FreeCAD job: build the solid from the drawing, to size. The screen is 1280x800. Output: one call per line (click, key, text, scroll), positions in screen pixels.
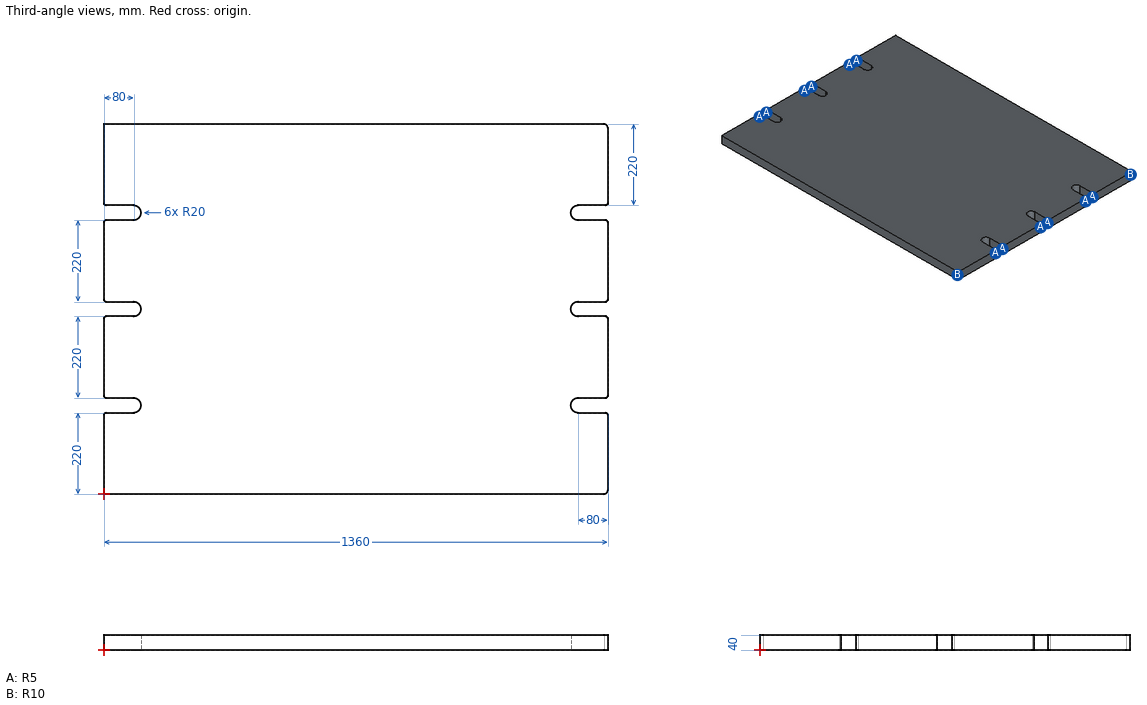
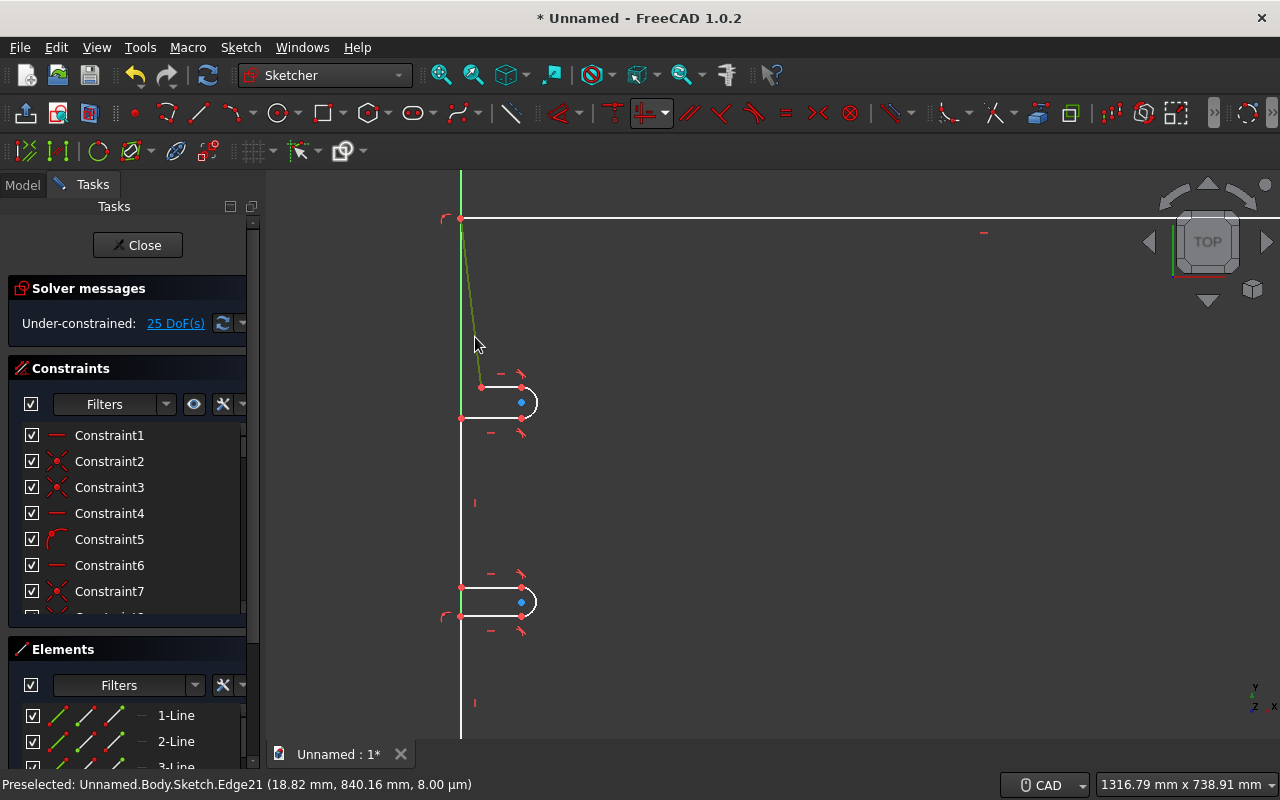
click(668, 114)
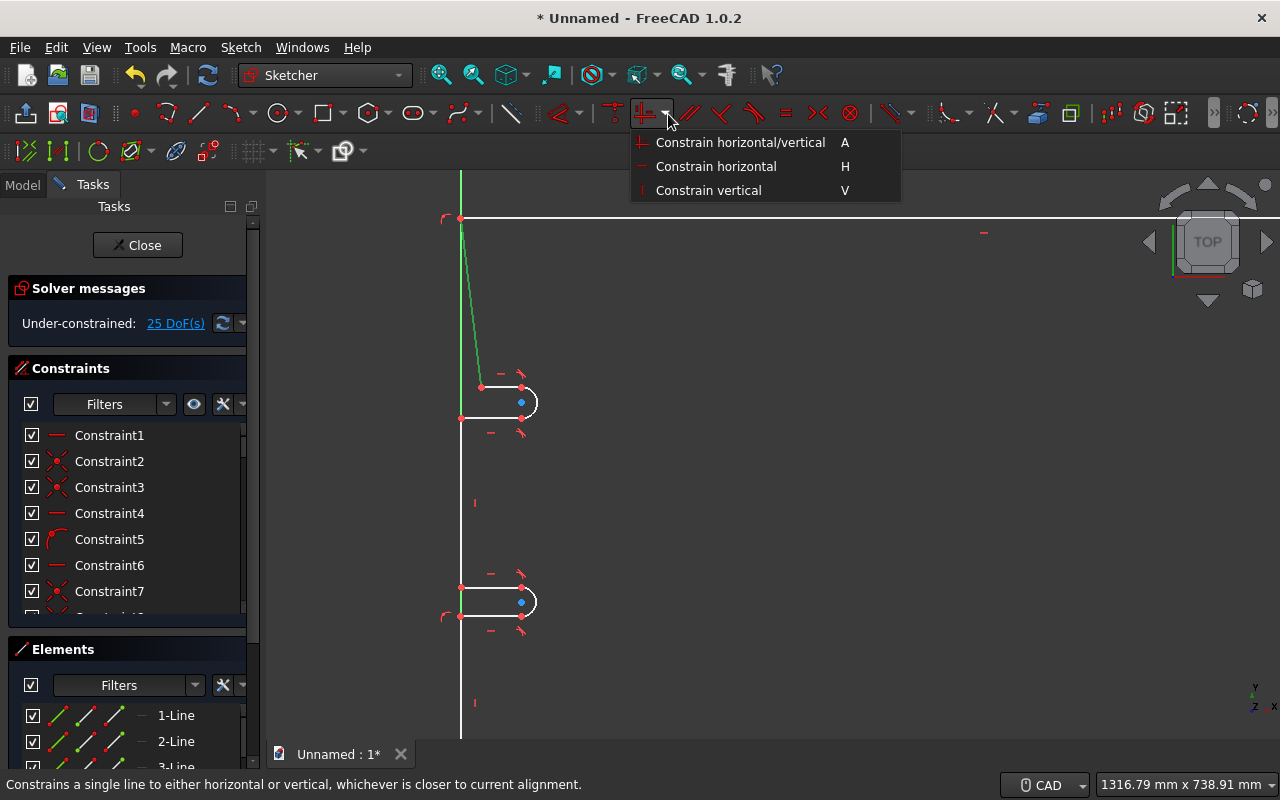
click(766, 190)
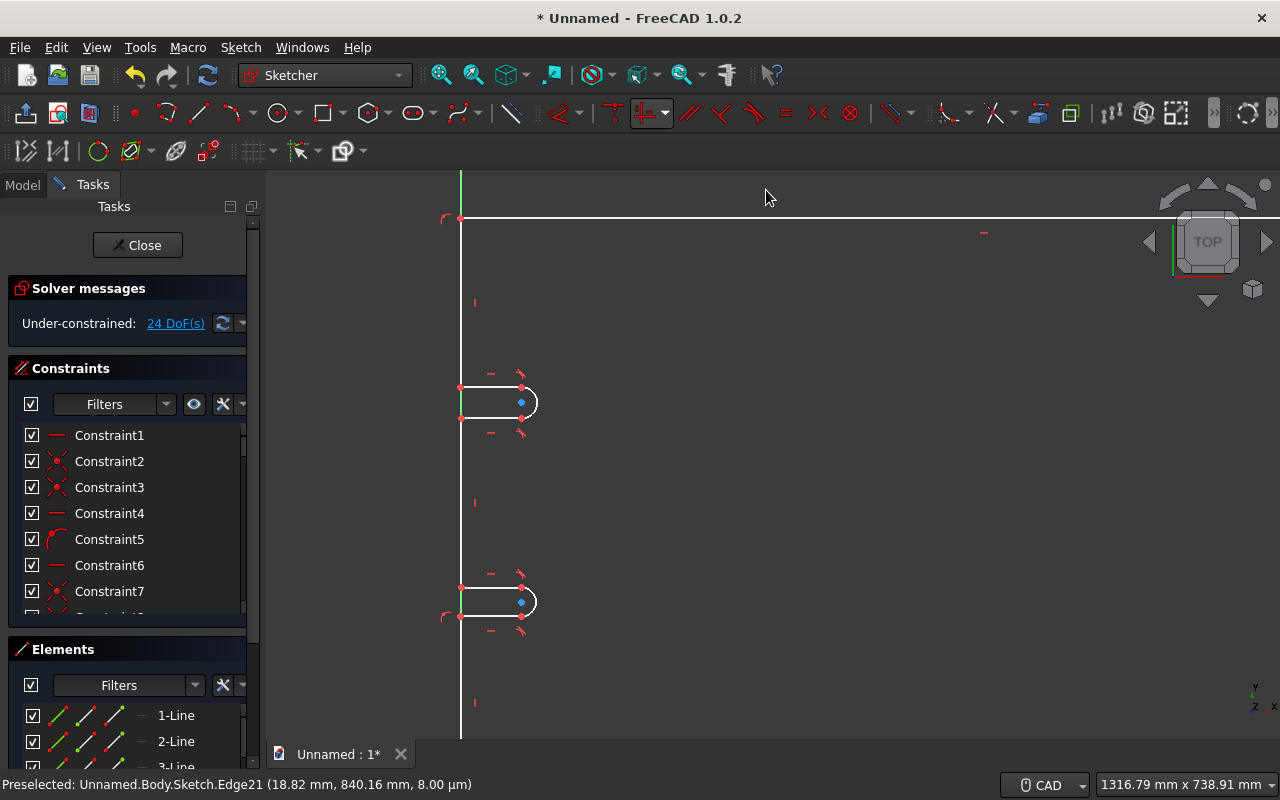
click(533, 611)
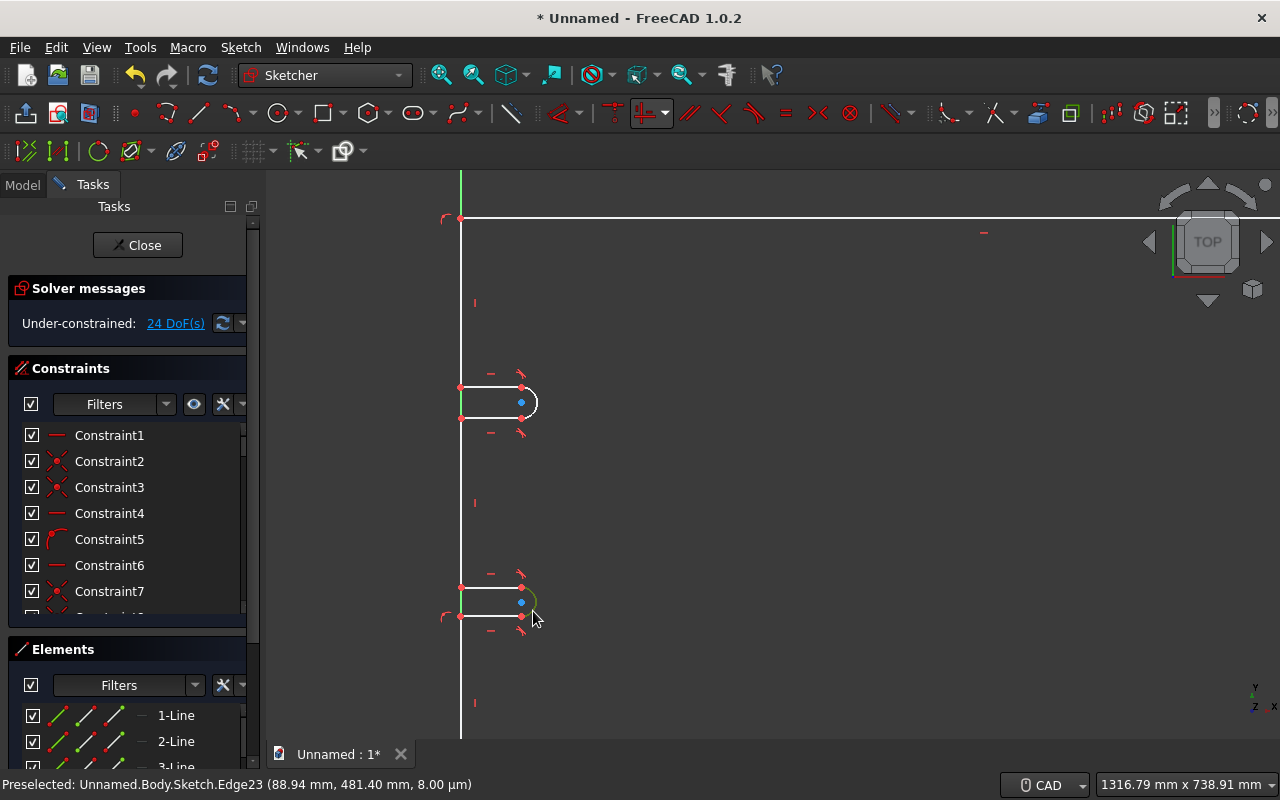
scroll(476, 336, down, 4)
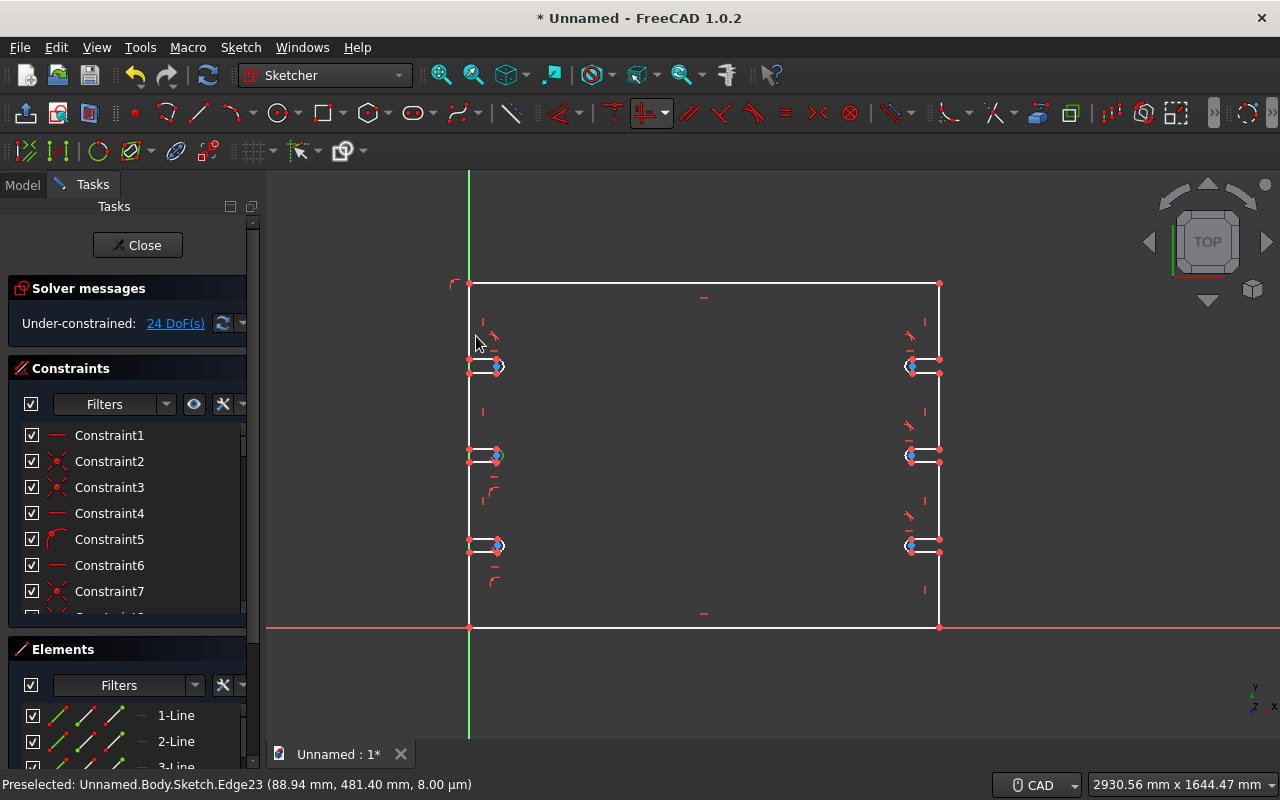
scroll(503, 550, up, 5)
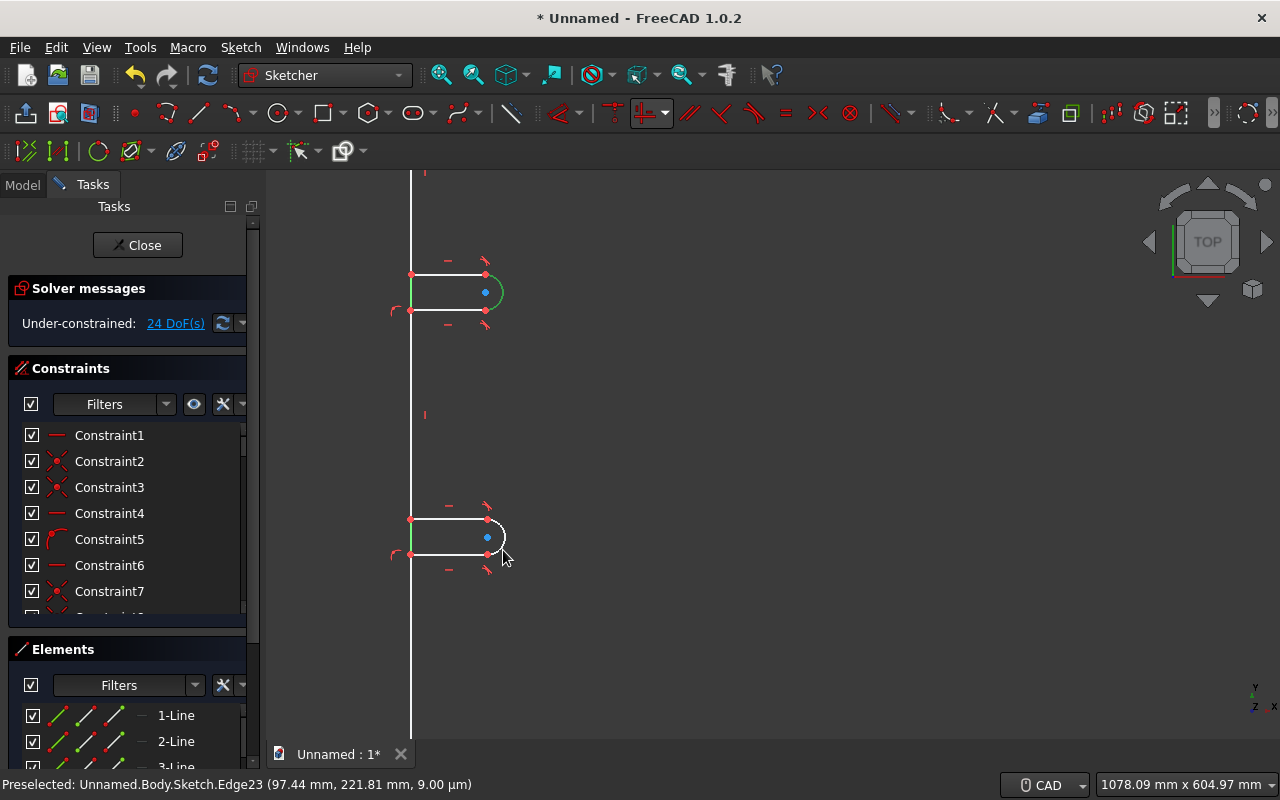
click(502, 548)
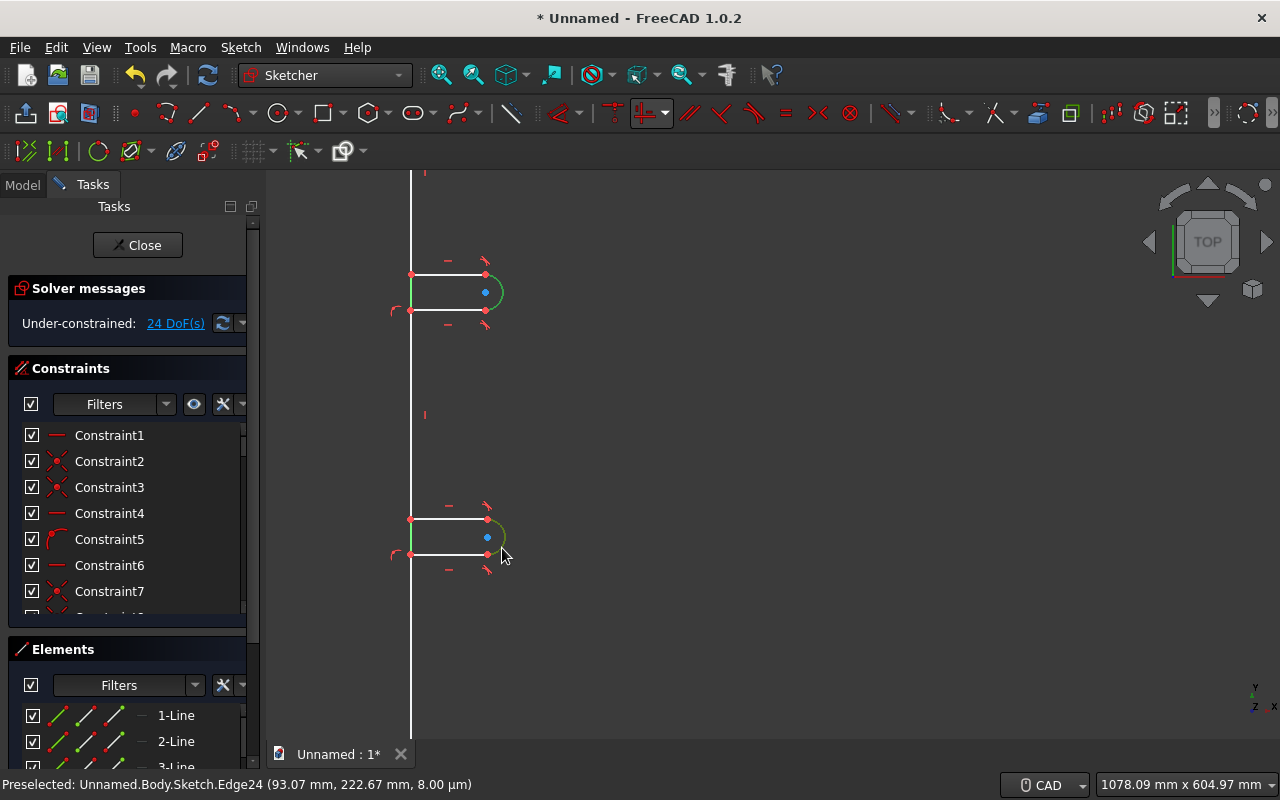
scroll(503, 550, down, 5)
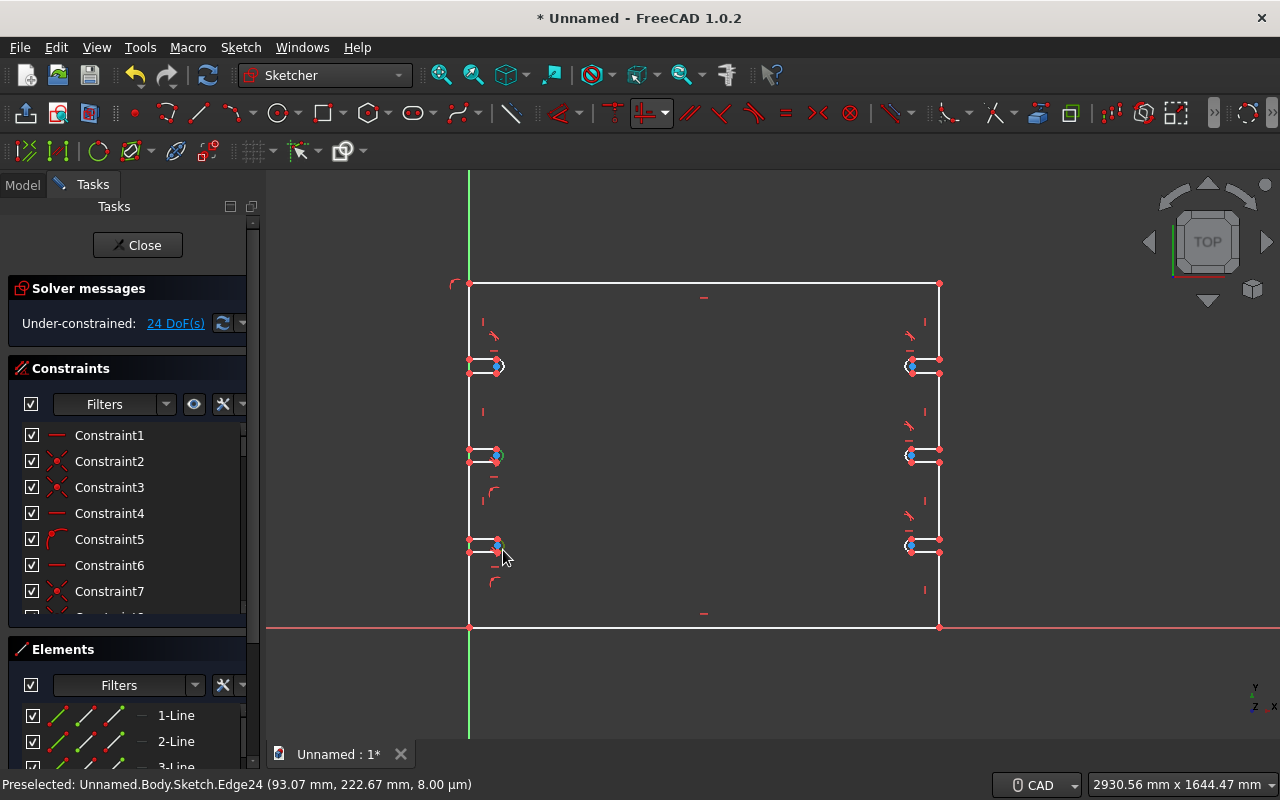
scroll(906, 542, up, 5)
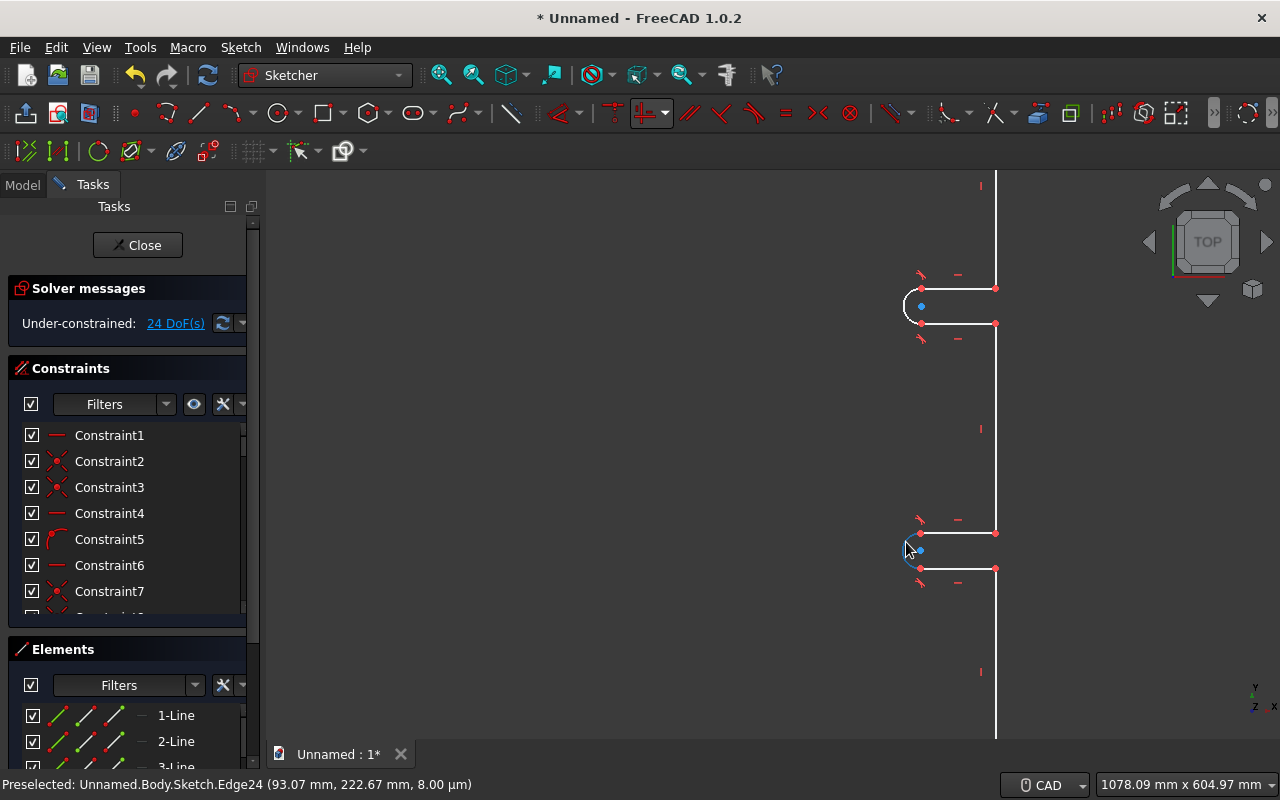
click(906, 541)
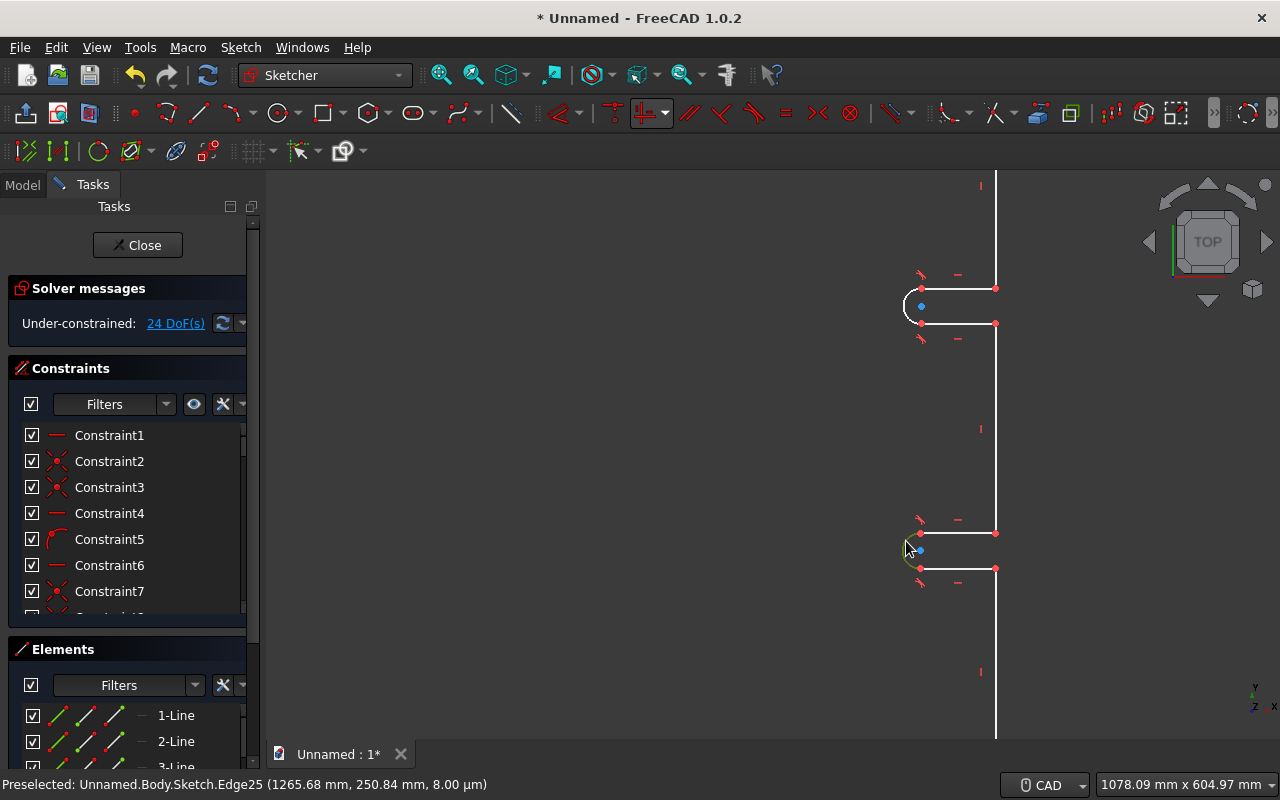
click(907, 296)